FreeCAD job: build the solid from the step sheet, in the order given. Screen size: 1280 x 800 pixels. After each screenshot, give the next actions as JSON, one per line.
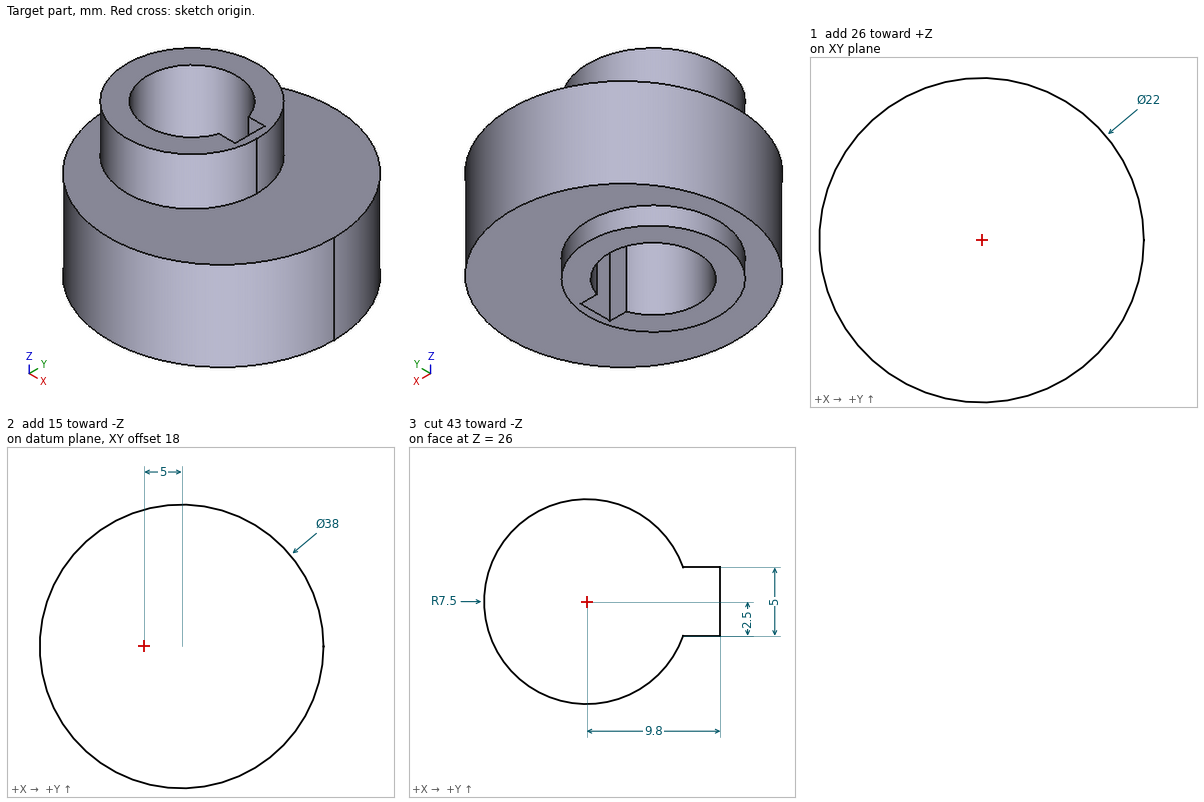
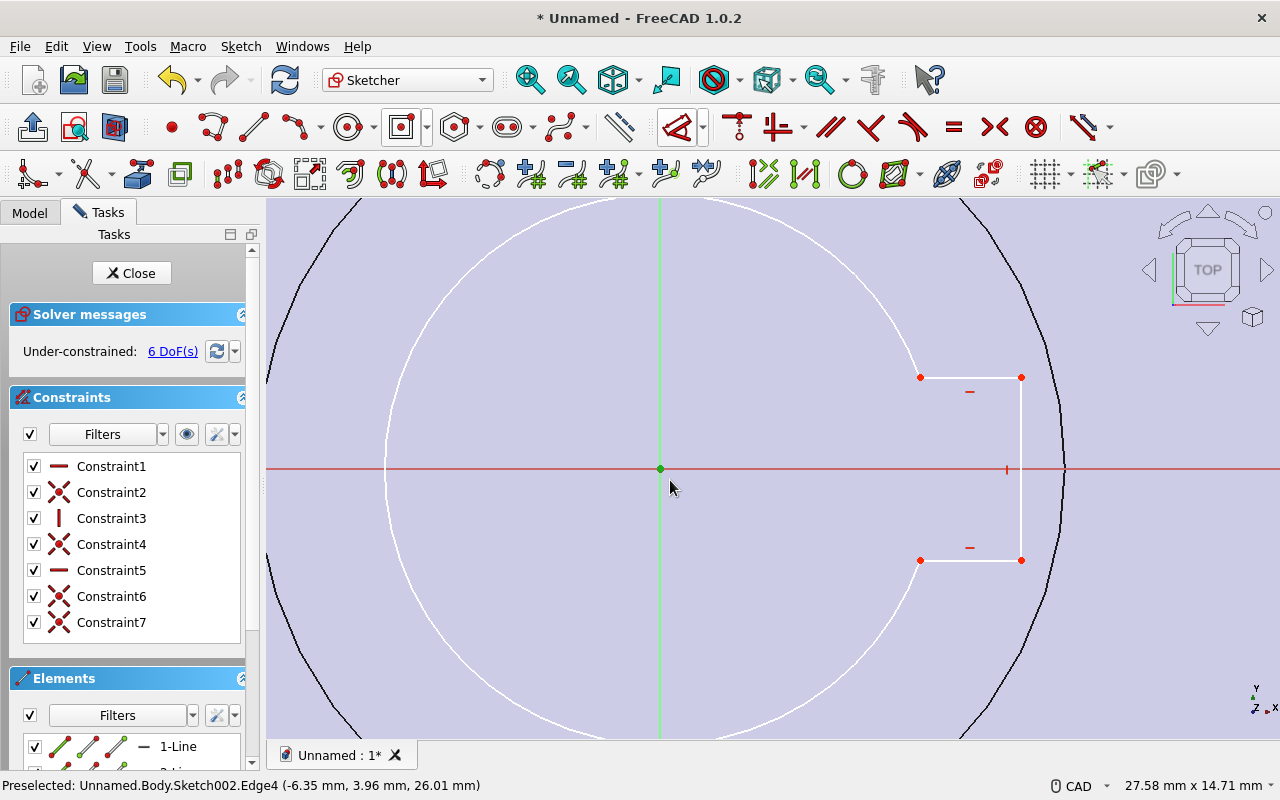
{"action": "left_click", "coordinate": [737, 128]}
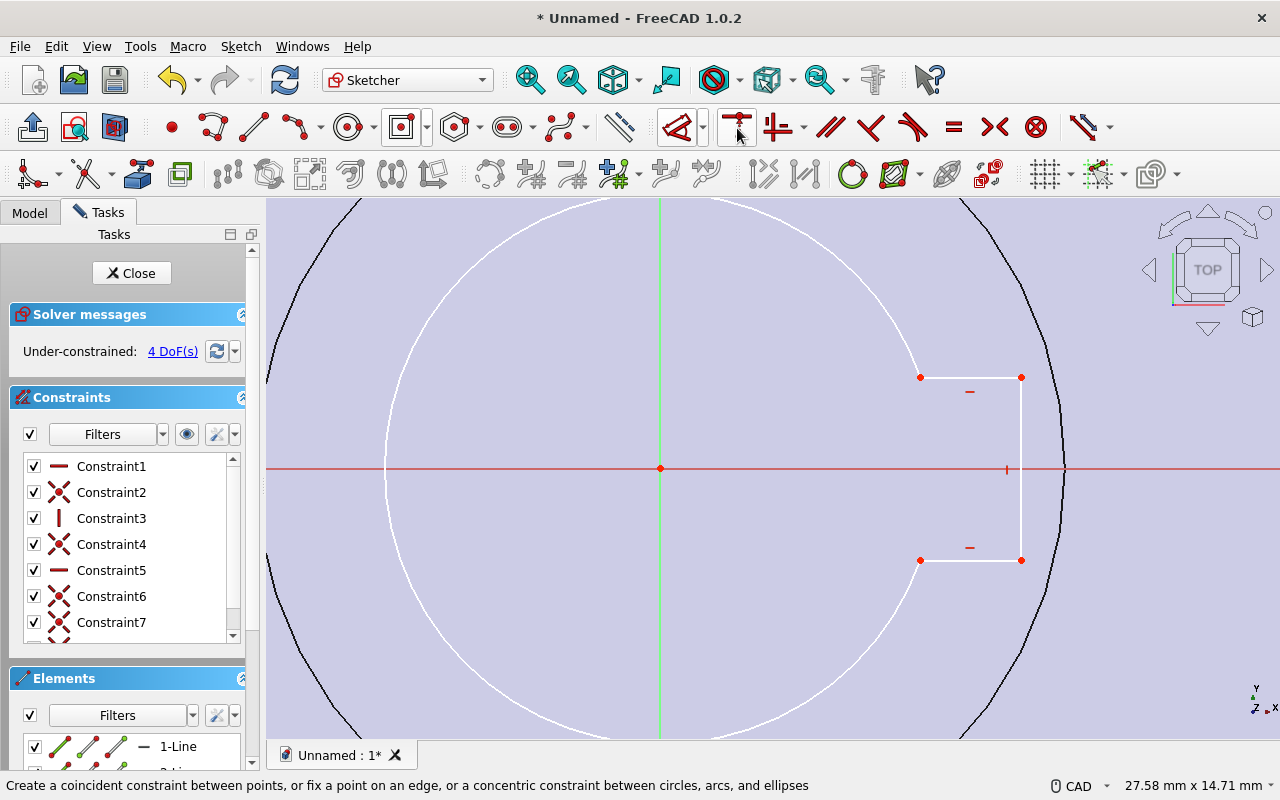
{"action": "key", "text": "d"}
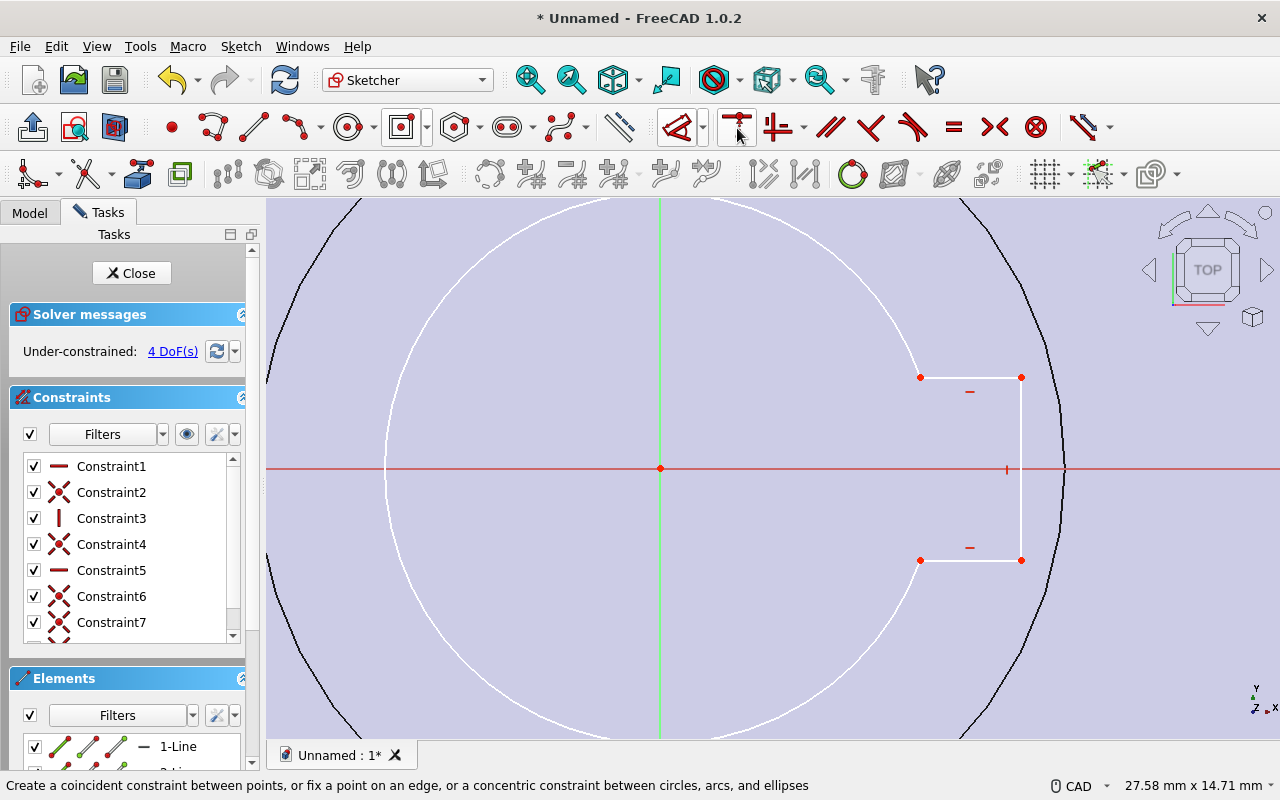
{"action": "left_click", "coordinate": [385, 467]}
{"action": "left_click", "coordinate": [391, 320]}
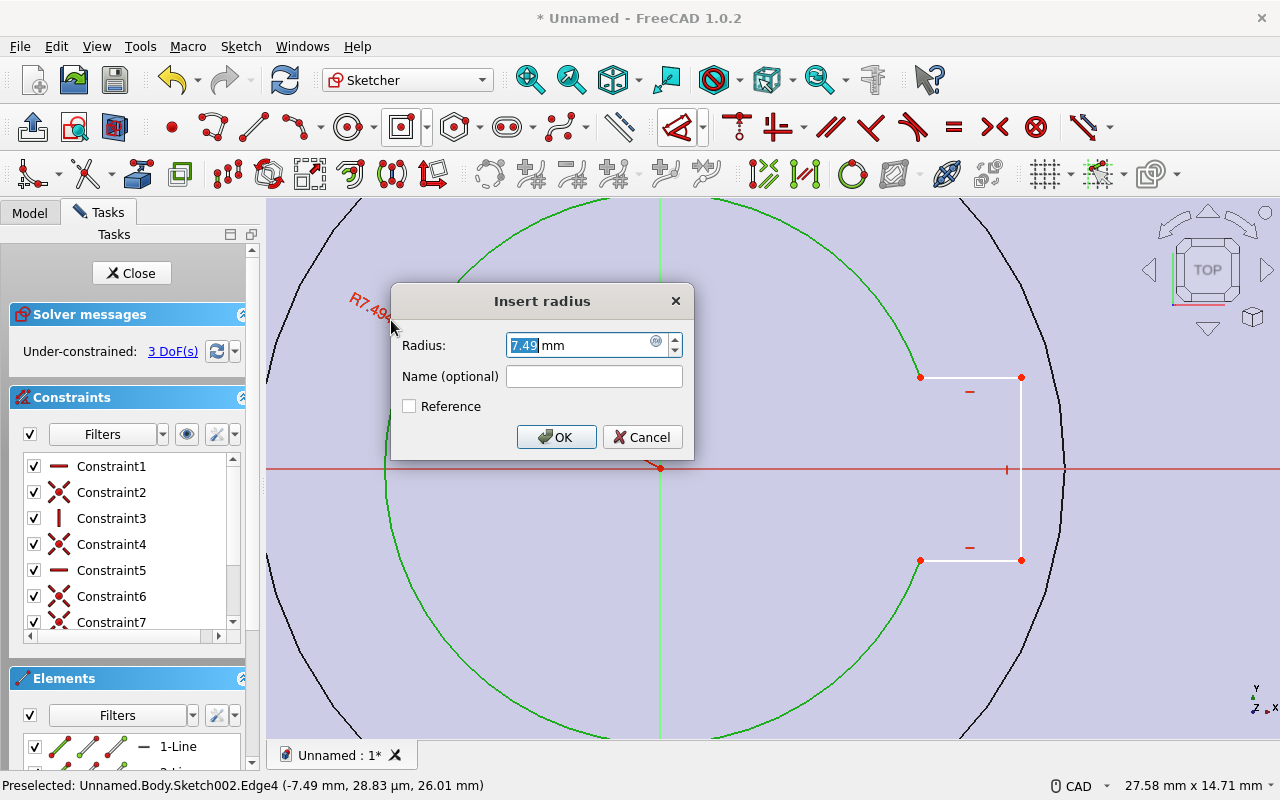
{"action": "type", "text": "7.5"}
{"action": "key", "text": "Return"}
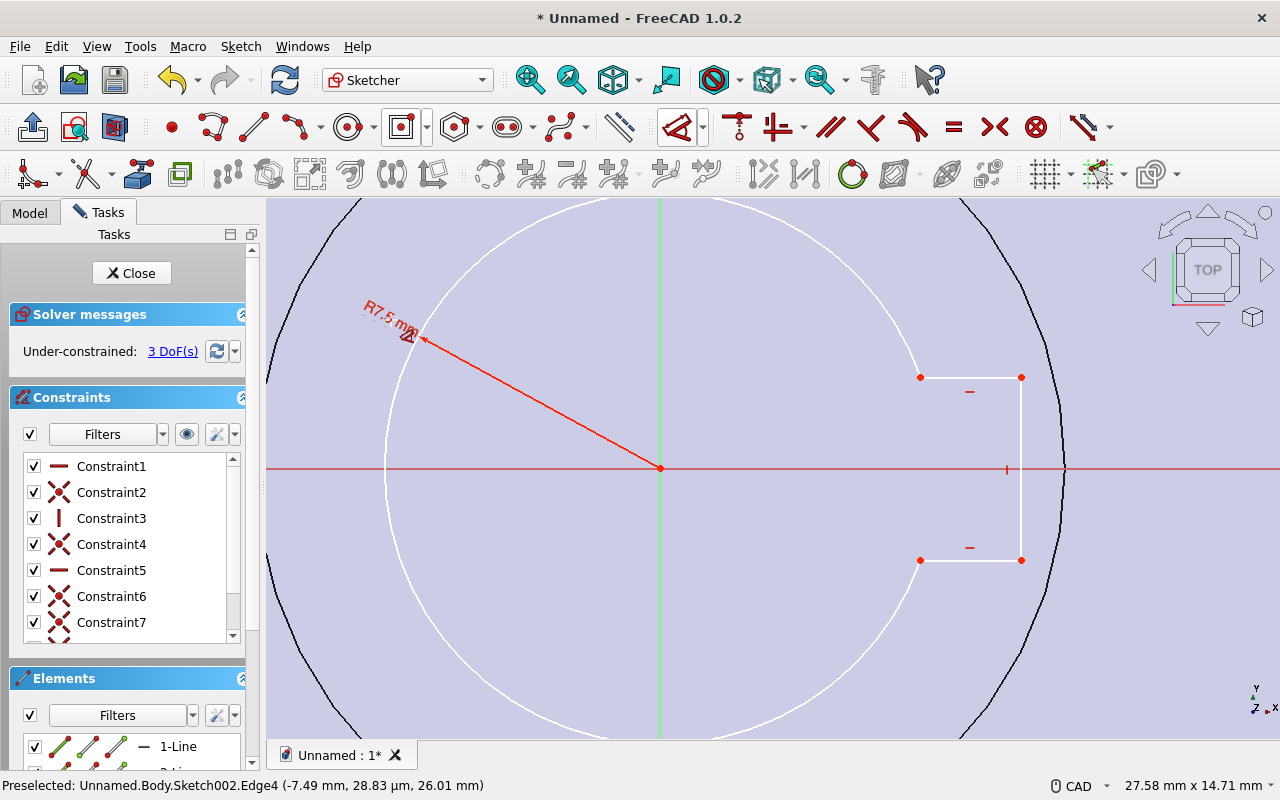
{"action": "left_click", "coordinate": [1021, 506]}
{"action": "left_click", "coordinate": [1055, 427]}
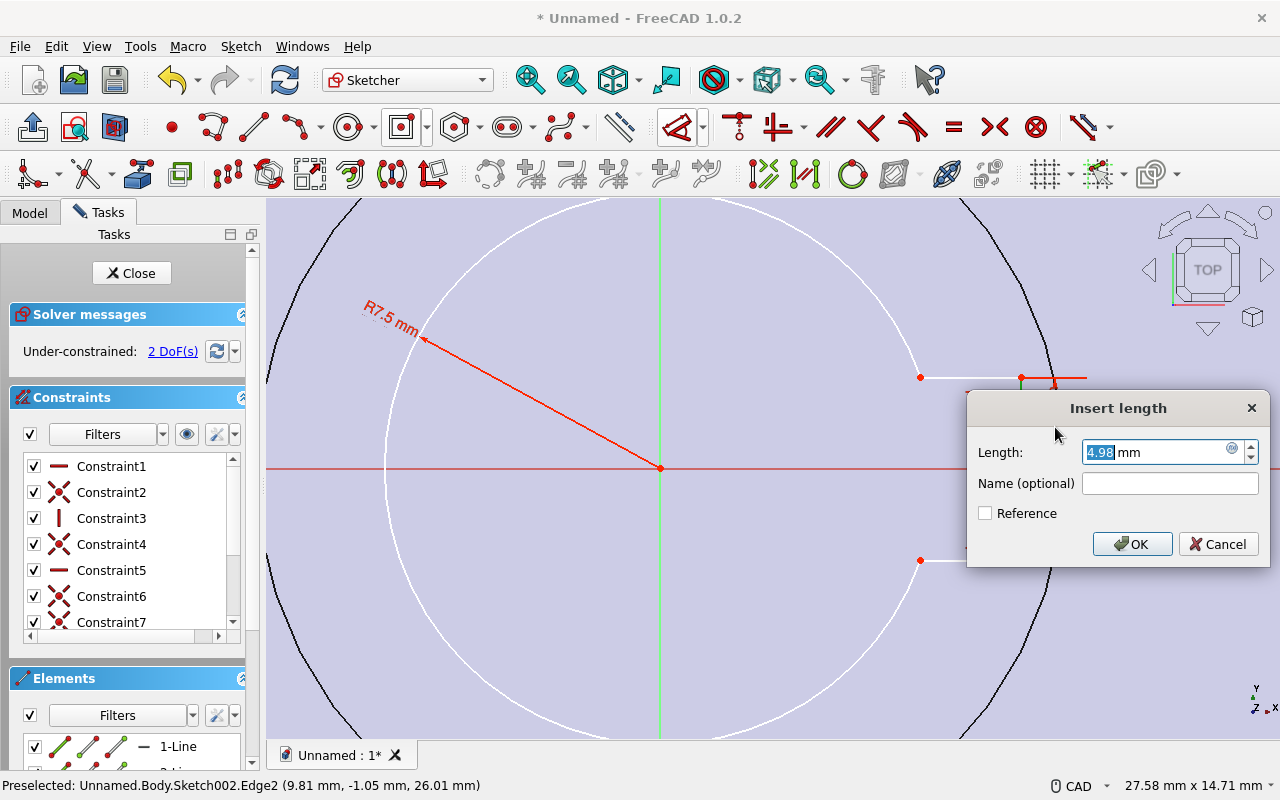
{"action": "type", "text": "5"}
{"action": "key", "text": "Return"}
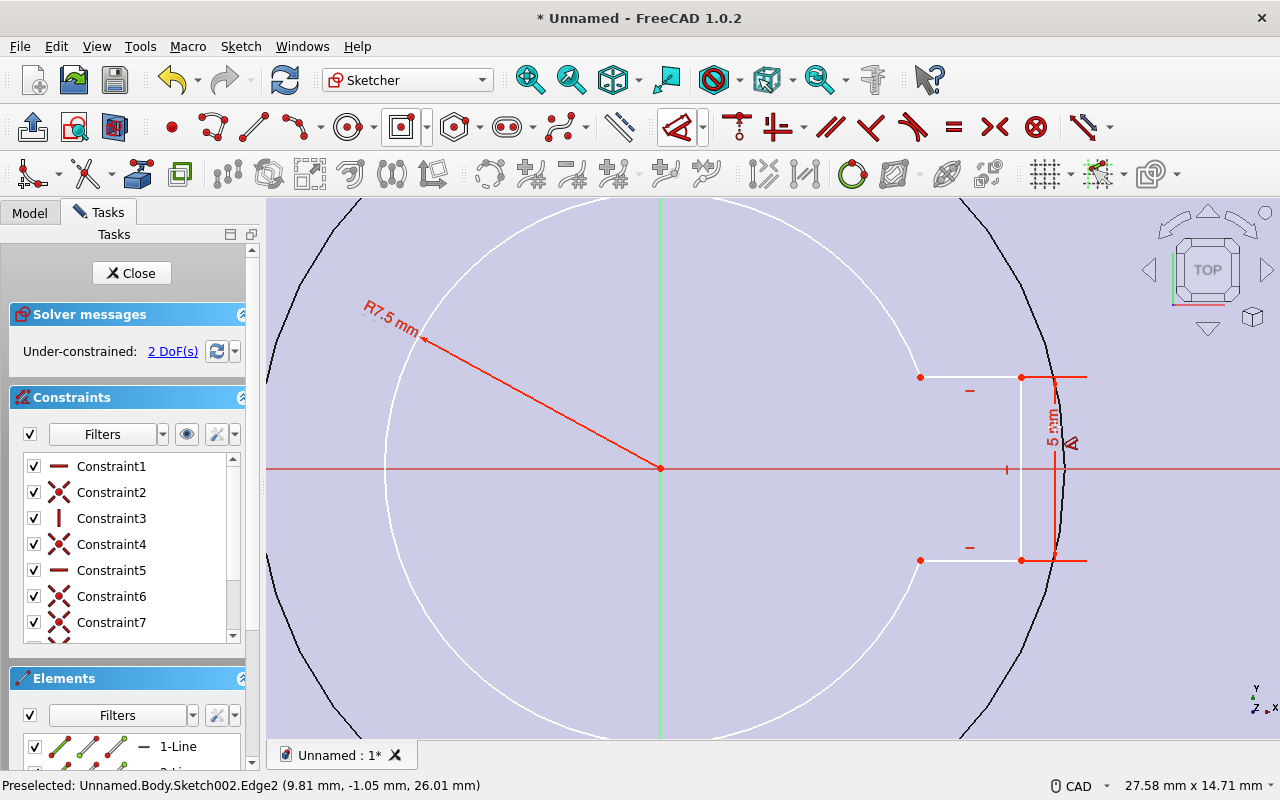
{"action": "left_click", "coordinate": [920, 561]}
{"action": "left_click", "coordinate": [954, 515]}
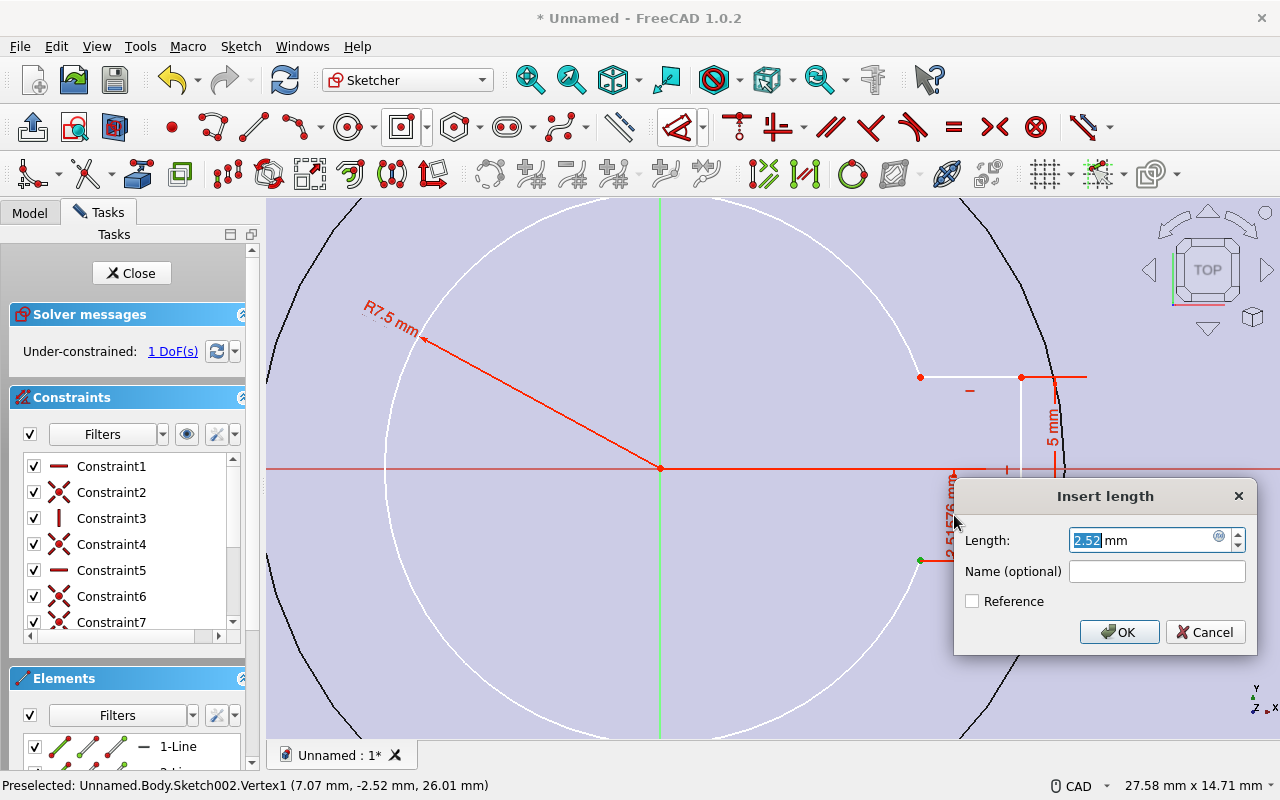
{"action": "type", "text": "2.5"}
{"action": "key", "text": "Return"}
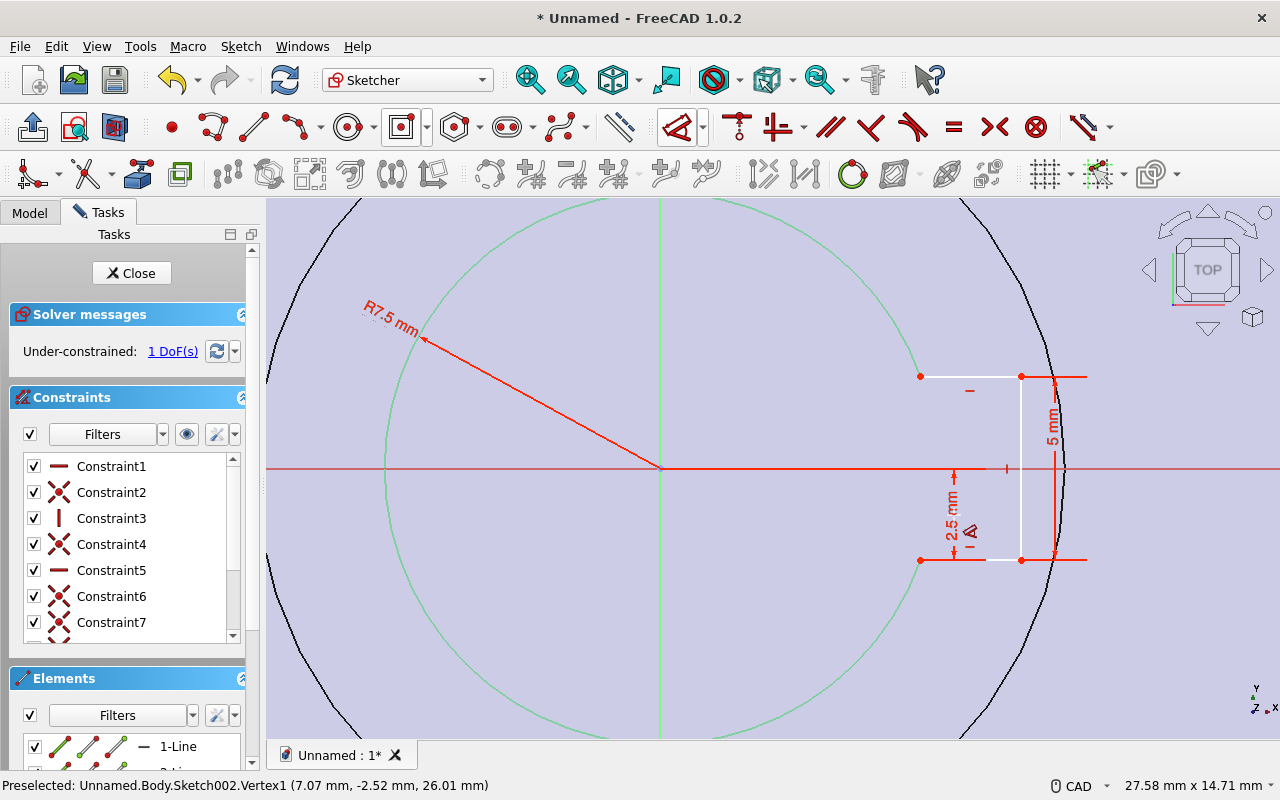
{"action": "left_click", "coordinate": [1021, 560]}
{"action": "left_click", "coordinate": [841, 594]}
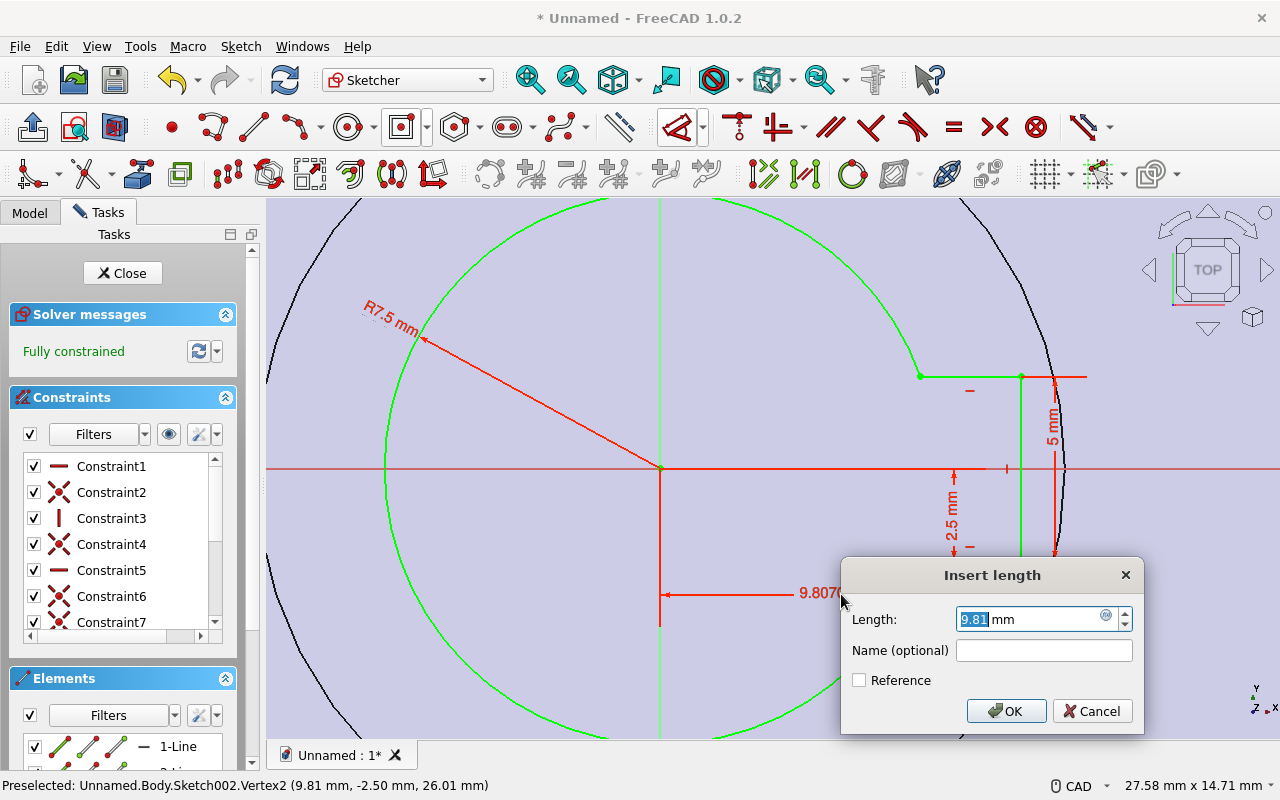
{"action": "type", "text": "9.8"}
{"action": "key", "text": "Return"}
{"action": "key", "text": "Escape"}